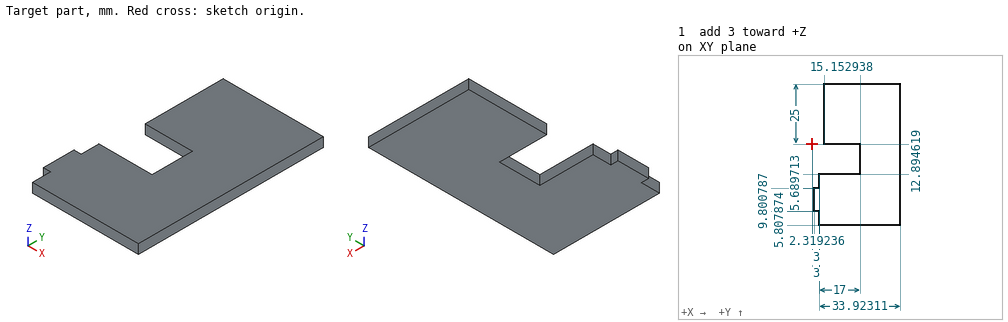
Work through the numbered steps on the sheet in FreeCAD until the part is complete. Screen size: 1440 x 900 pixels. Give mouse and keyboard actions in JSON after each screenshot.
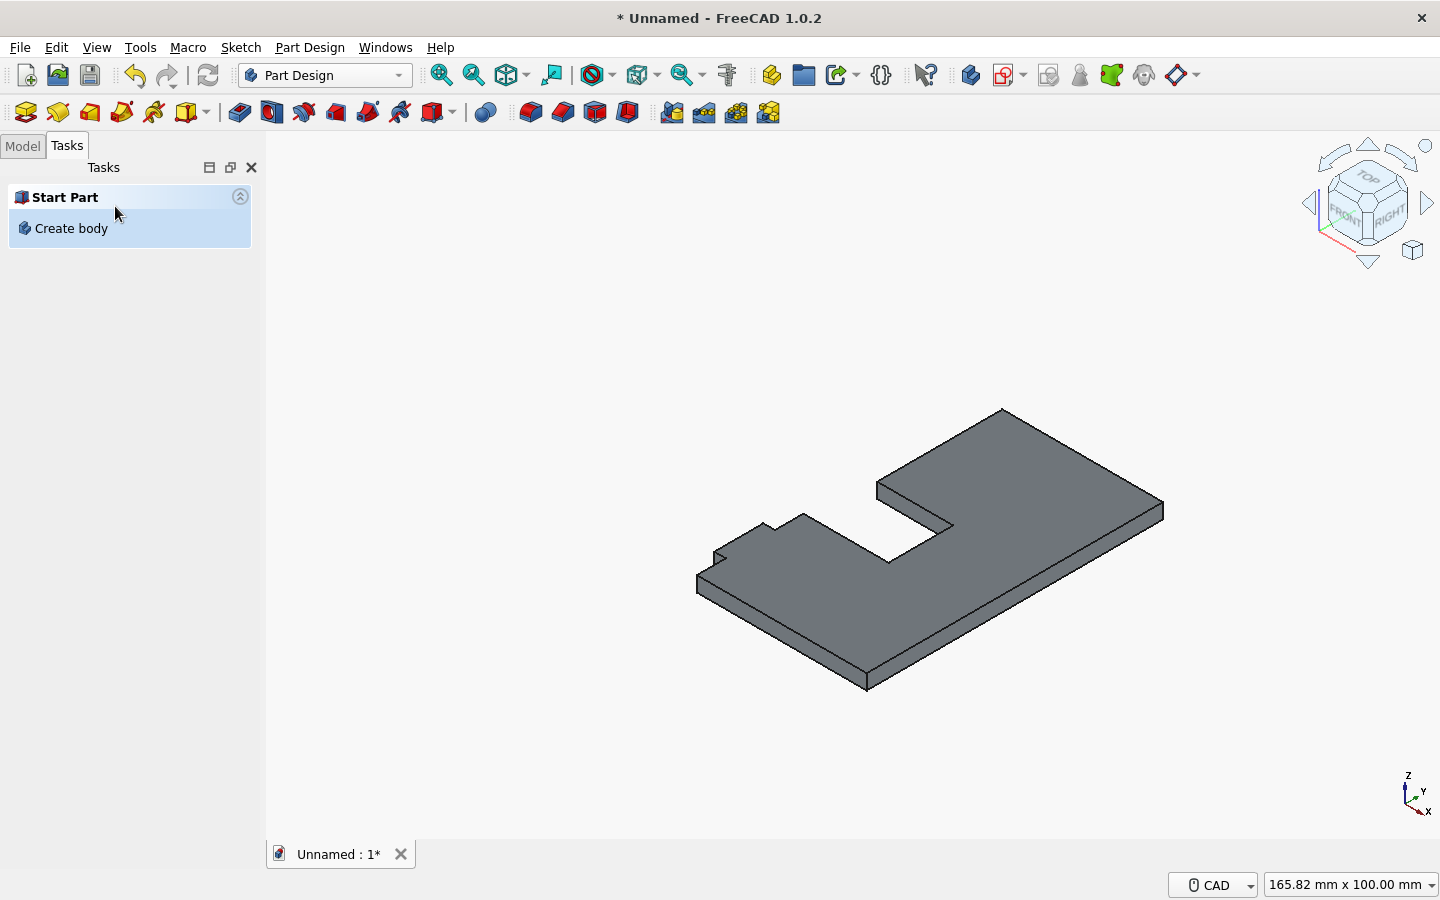
{"action": "left_click", "coordinate": [442, 76]}